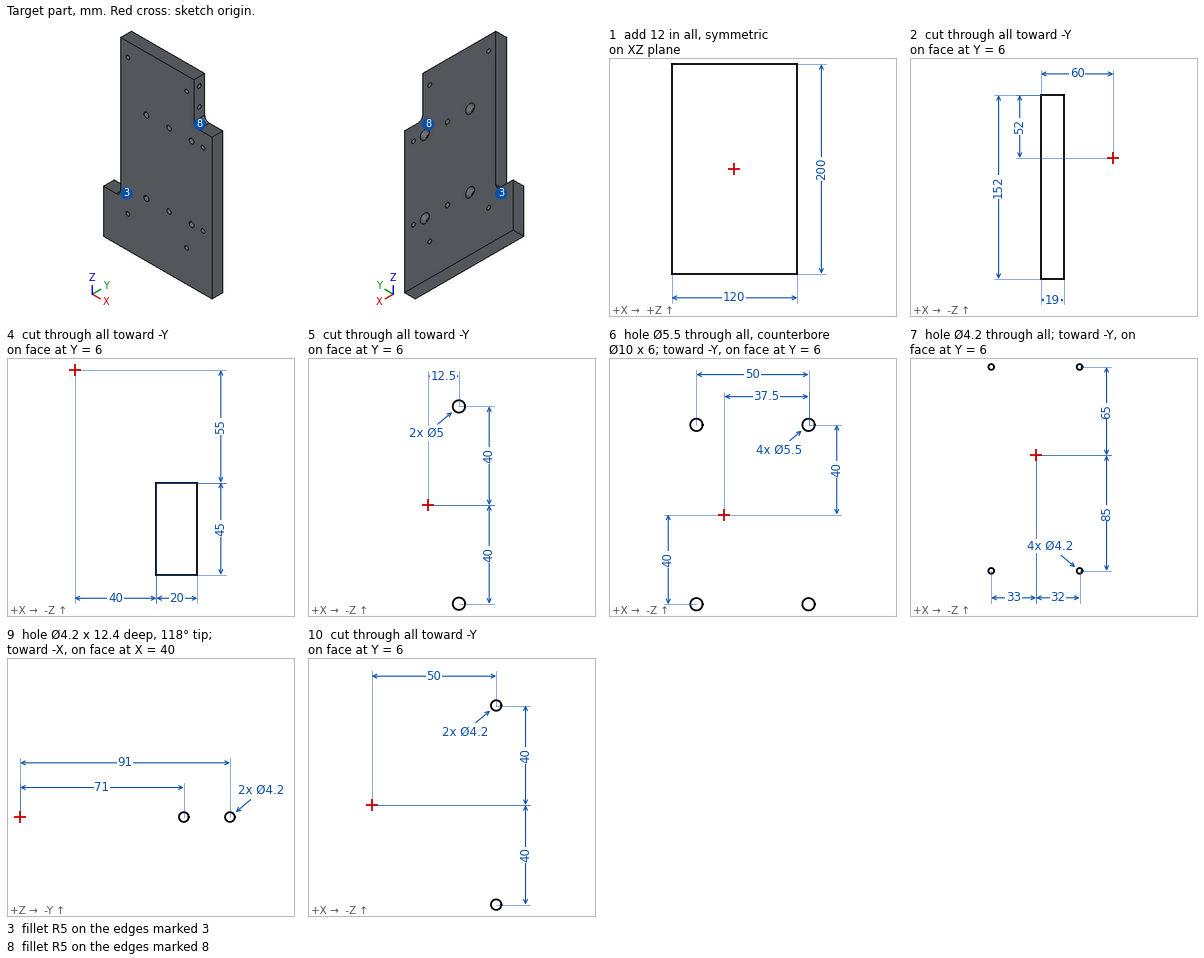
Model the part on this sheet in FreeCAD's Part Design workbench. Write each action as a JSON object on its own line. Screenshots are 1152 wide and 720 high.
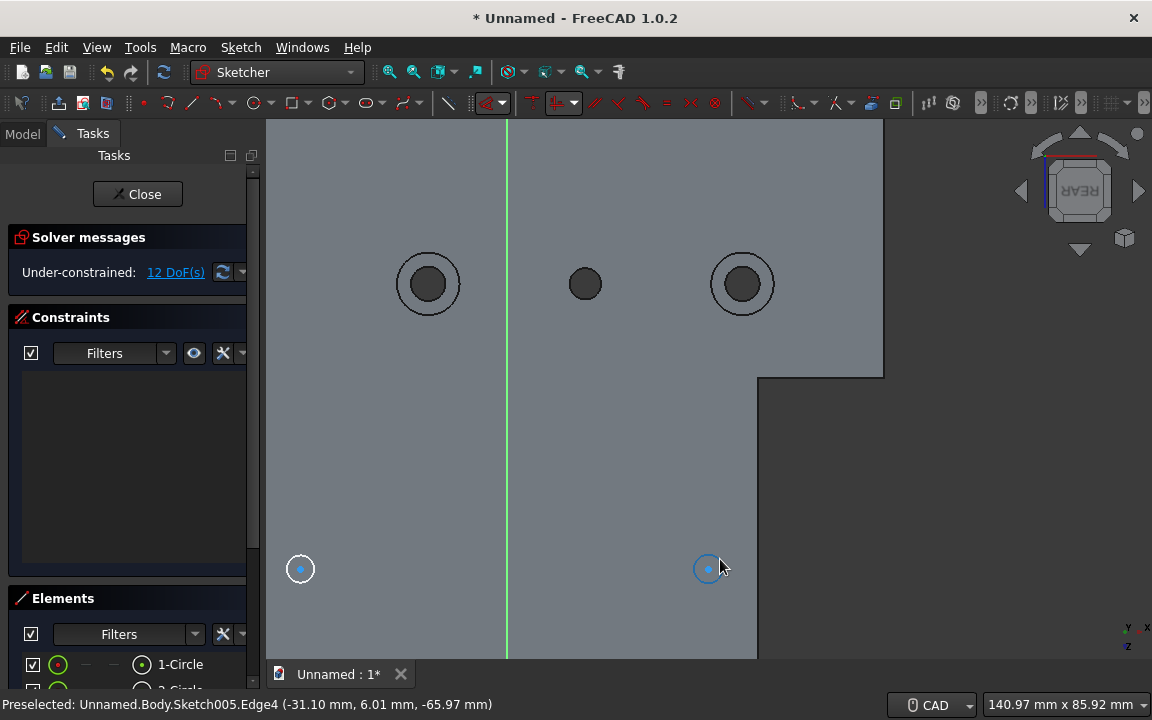
{"action": "left_click", "coordinate": [718, 559]}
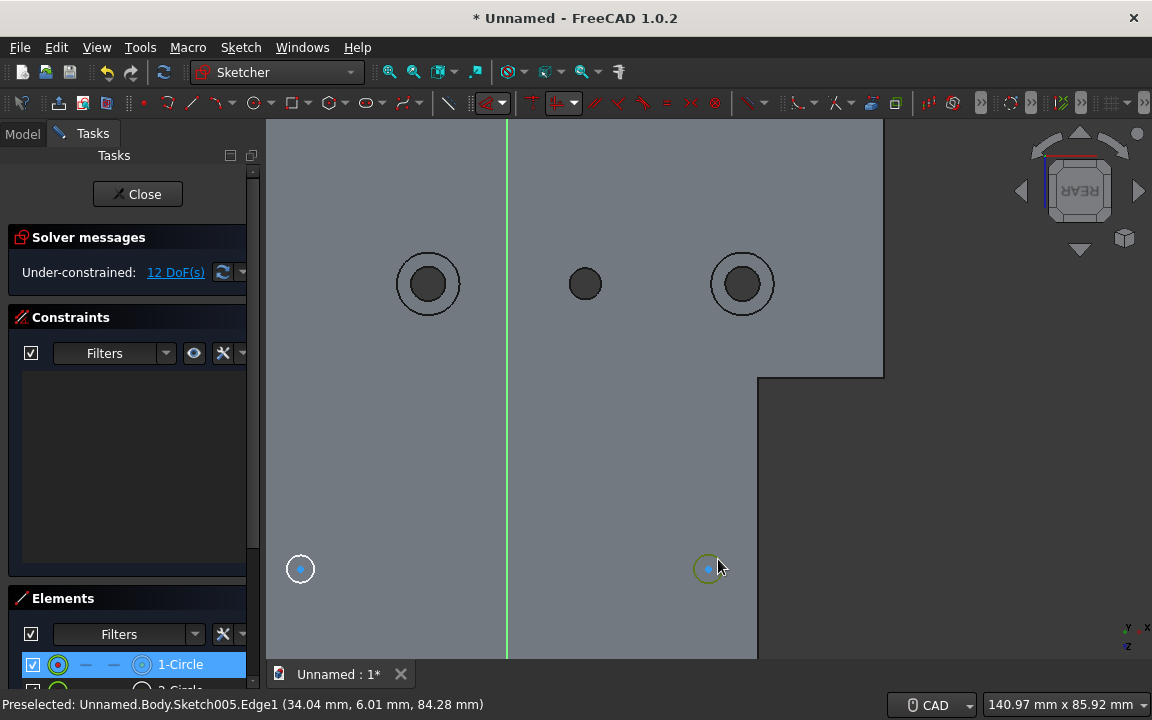
{"action": "left_click", "coordinate": [310, 559]}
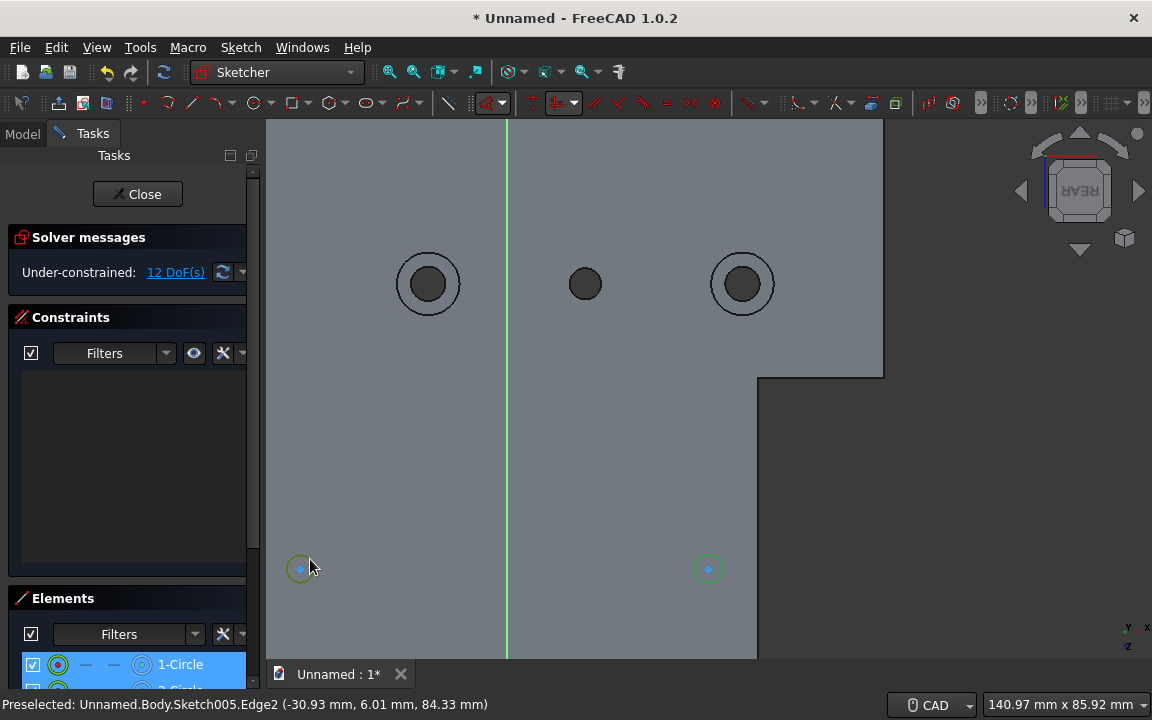
{"action": "scroll", "coordinate": [720, 560], "scroll_direction": "down", "scroll_amount": 5}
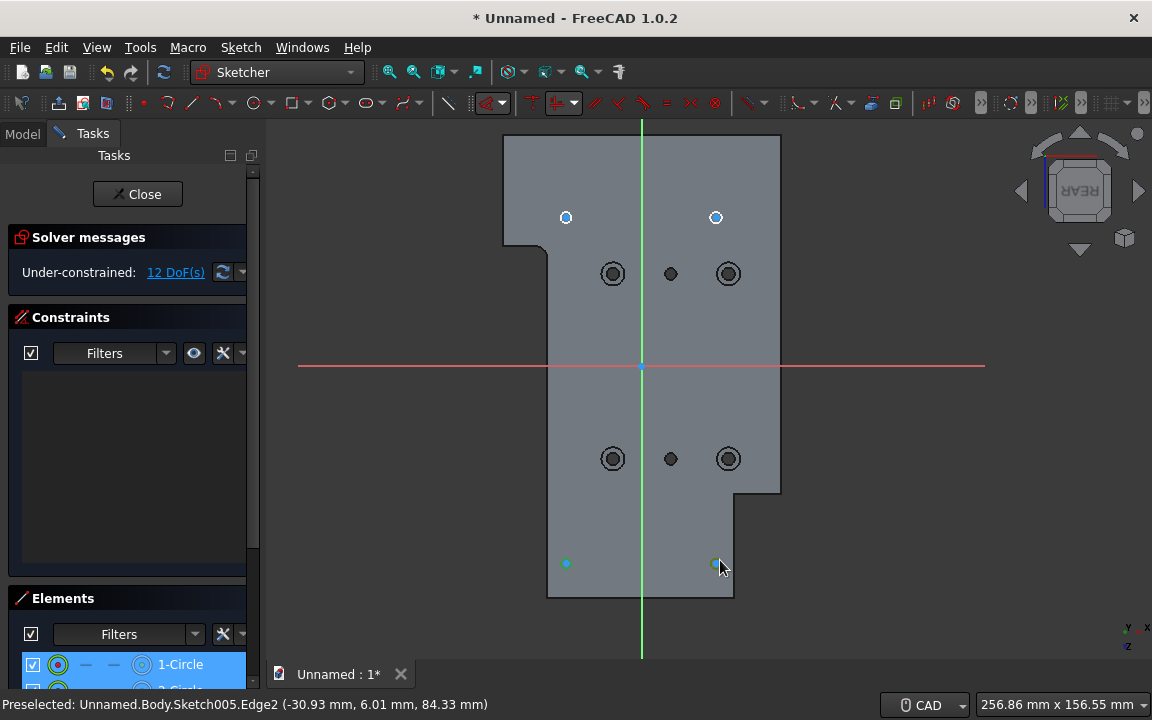
{"action": "scroll", "coordinate": [720, 214], "scroll_direction": "up", "scroll_amount": 5}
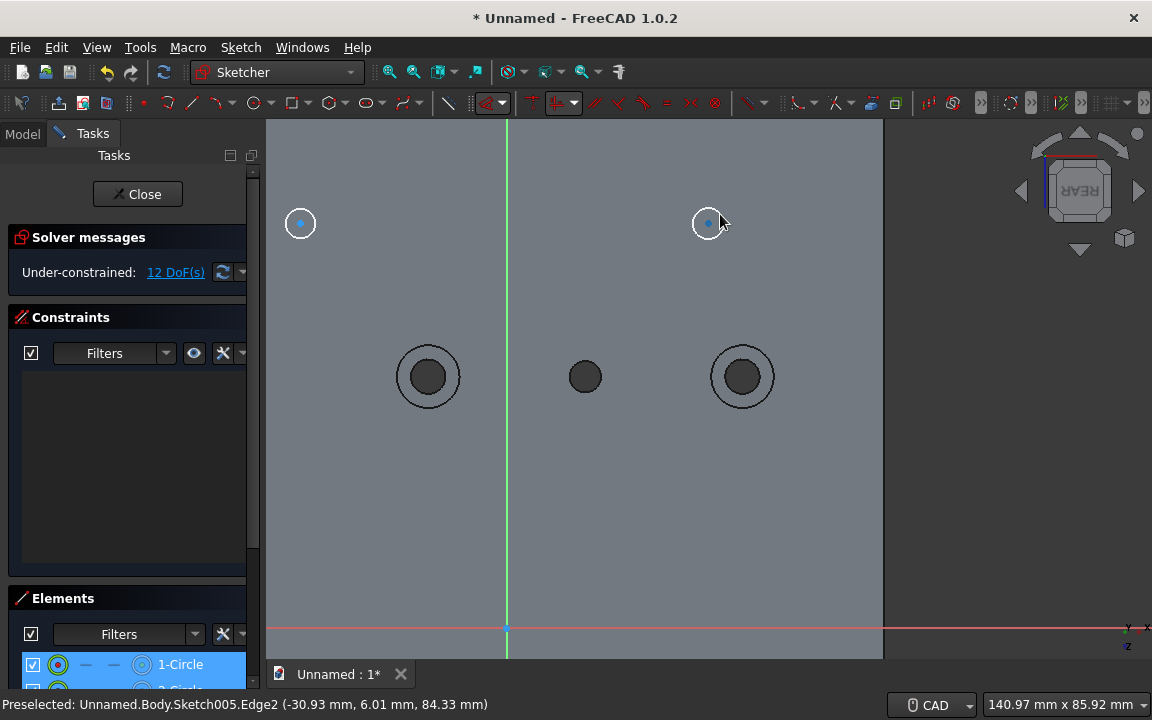
{"action": "left_click", "coordinate": [719, 213]}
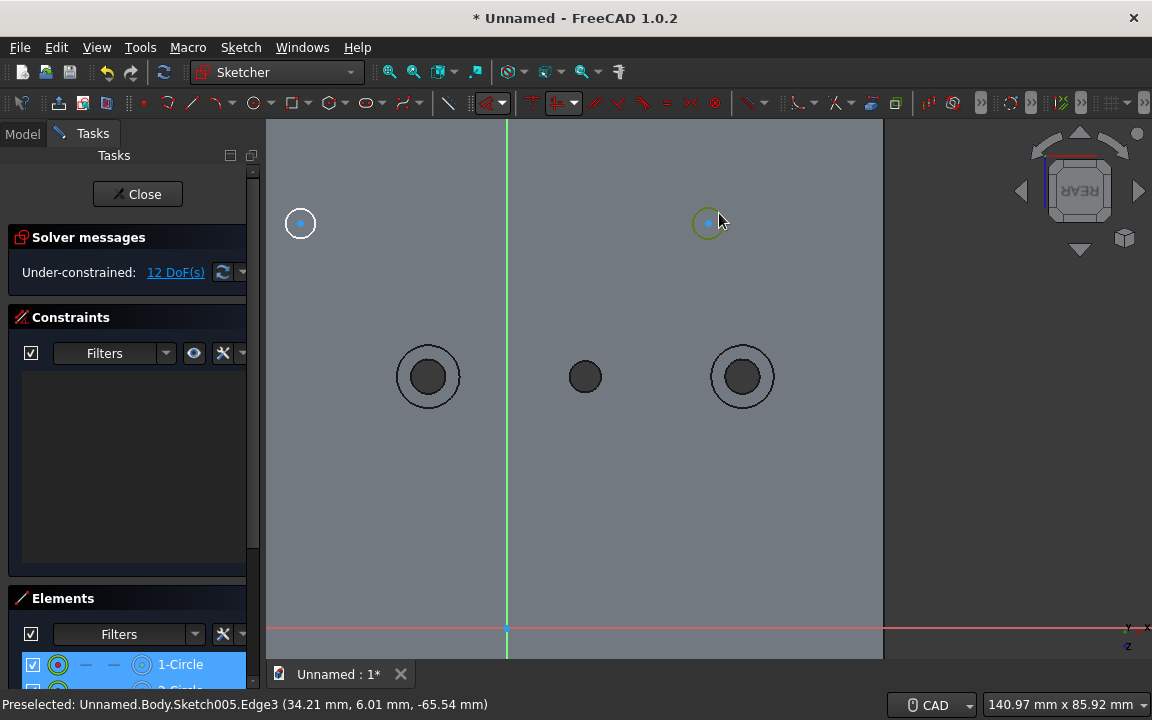
{"action": "left_click", "coordinate": [311, 213]}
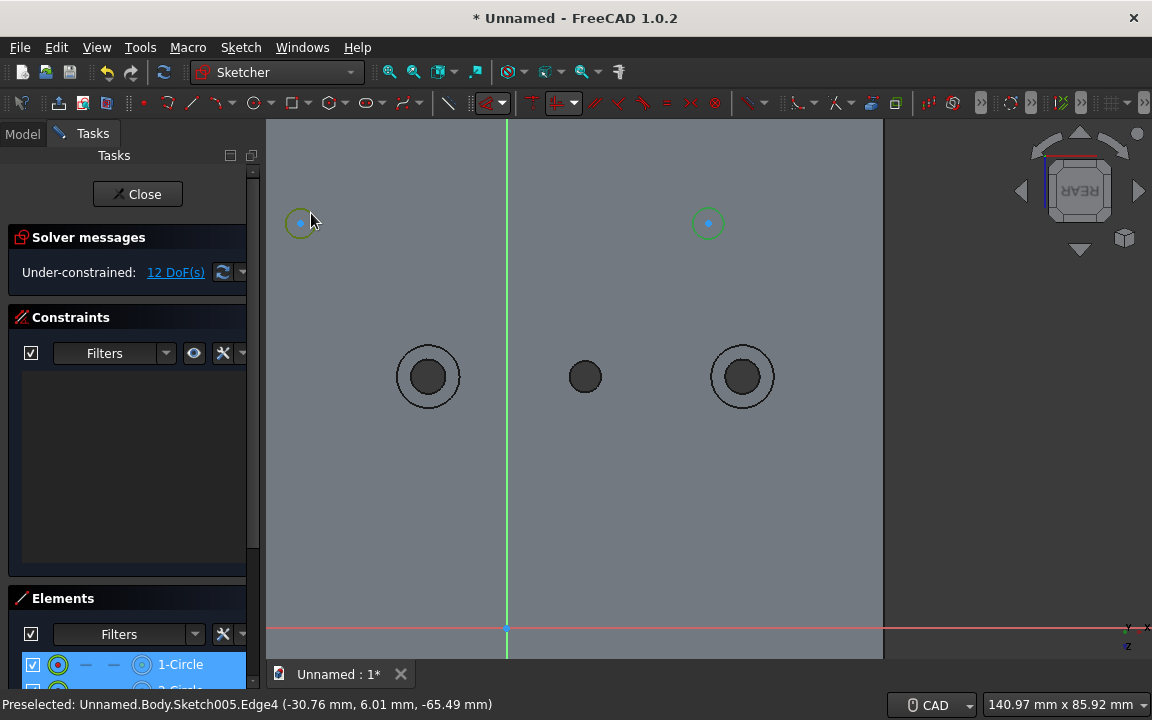
{"action": "left_click", "coordinate": [668, 104]}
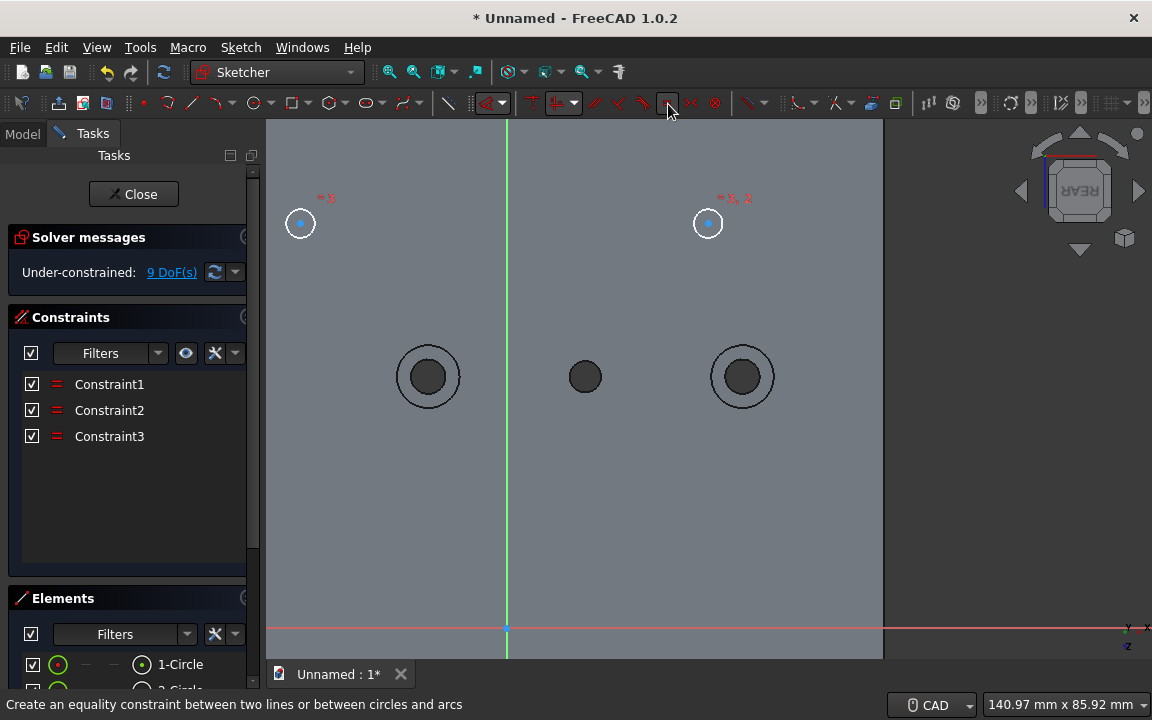
{"action": "scroll", "coordinate": [720, 213], "scroll_direction": "down", "scroll_amount": 5}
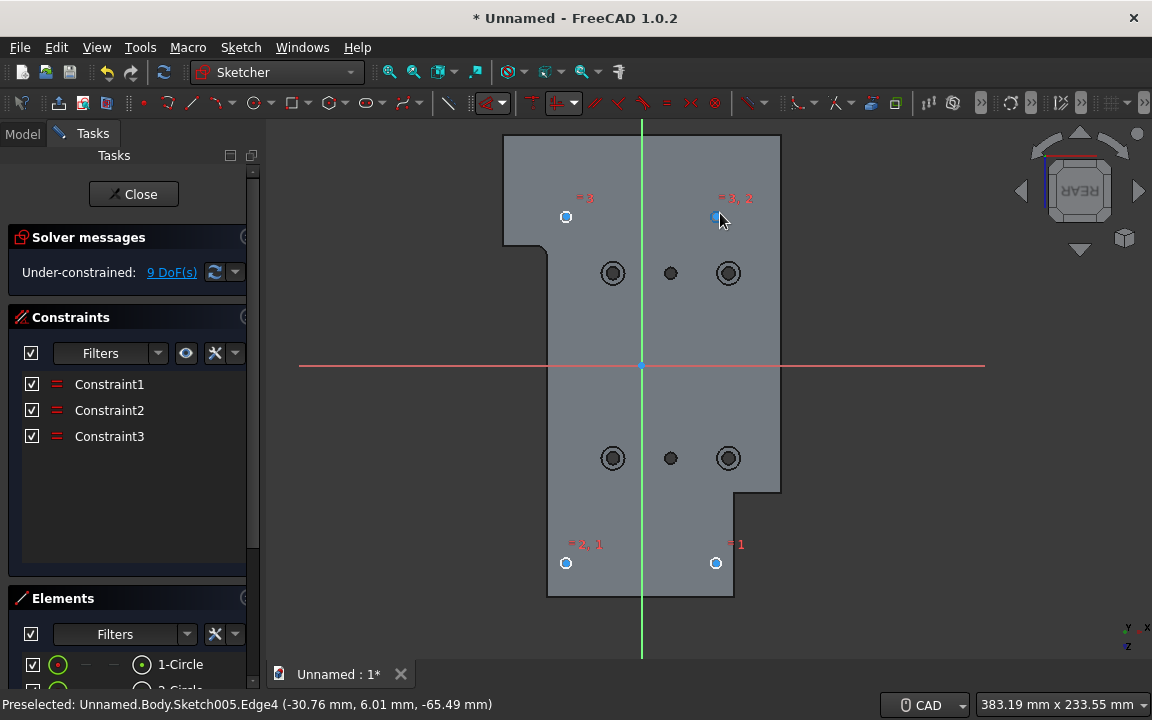
{"action": "left_click", "coordinate": [716, 563]}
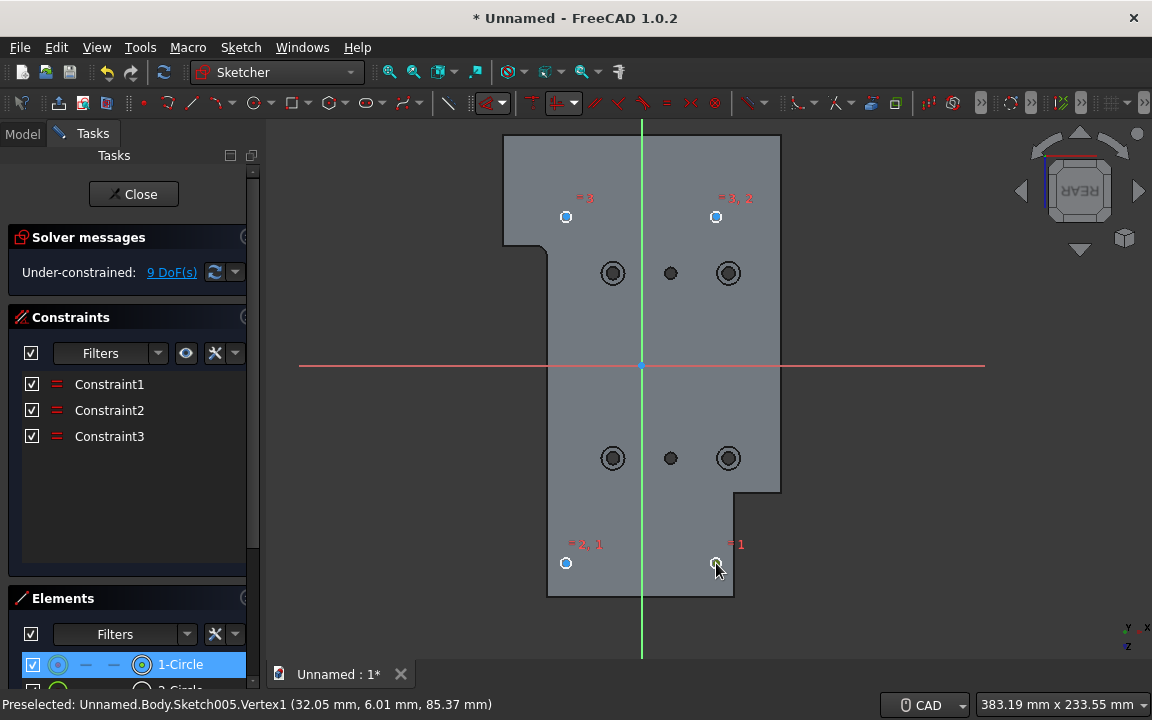
{"action": "left_click", "coordinate": [566, 563]}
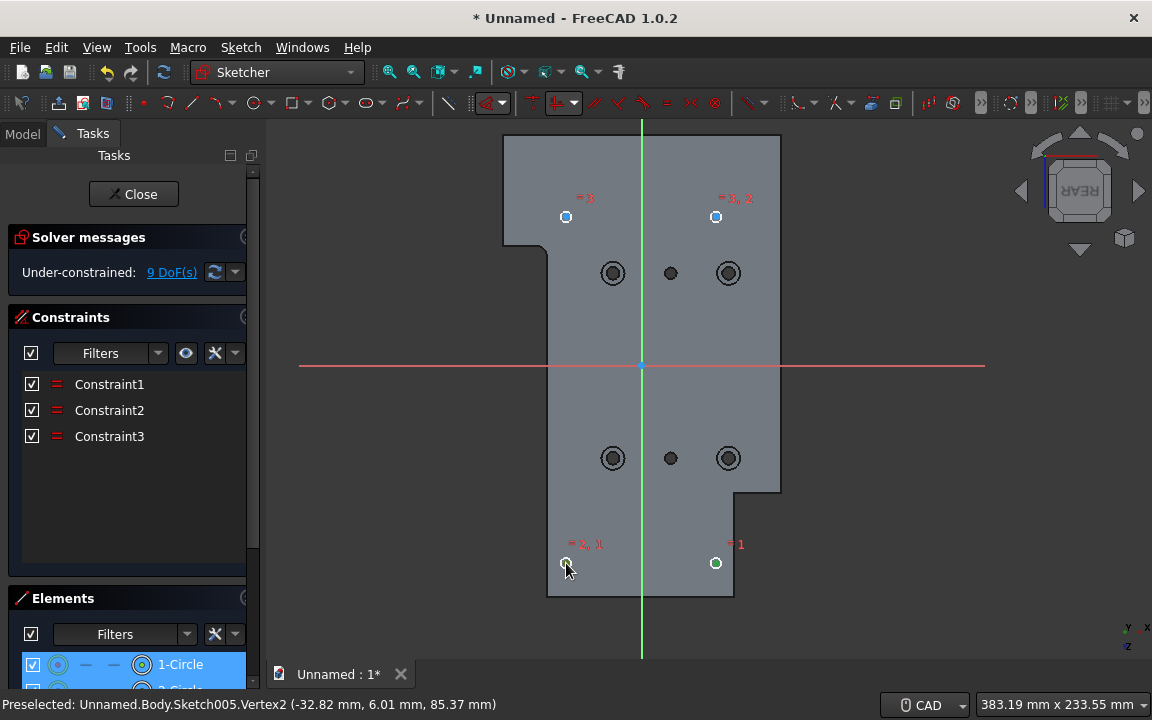
{"action": "left_click", "coordinate": [576, 104]}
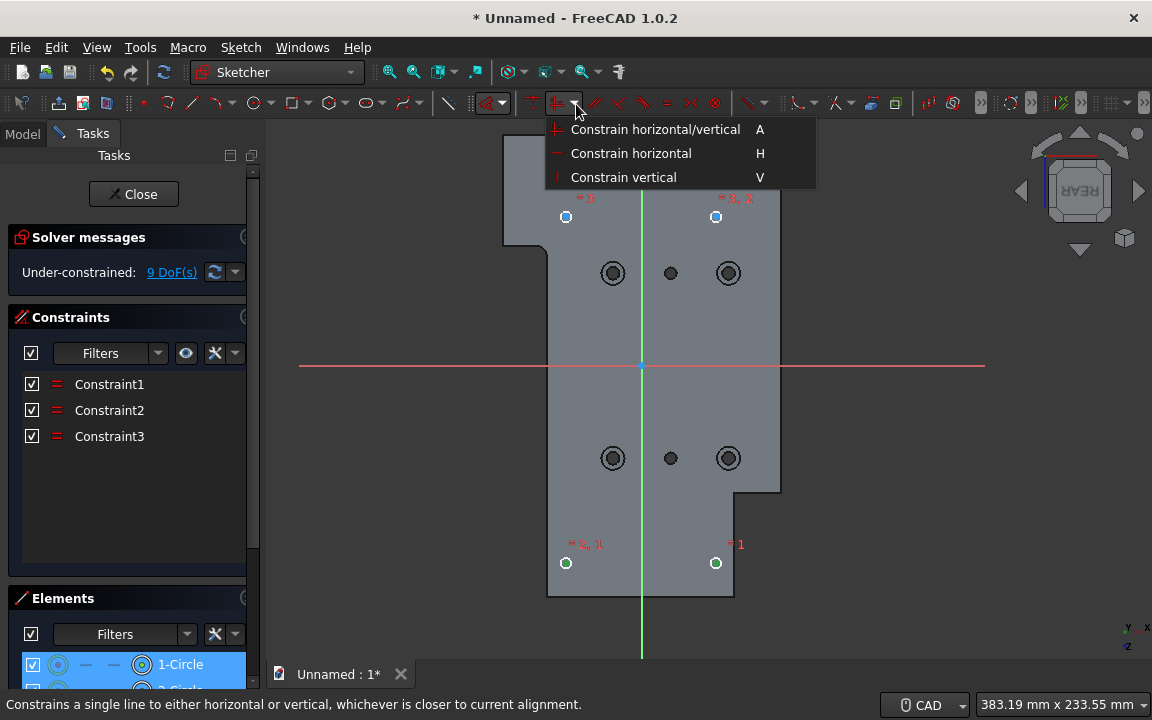
{"action": "left_click", "coordinate": [681, 153]}